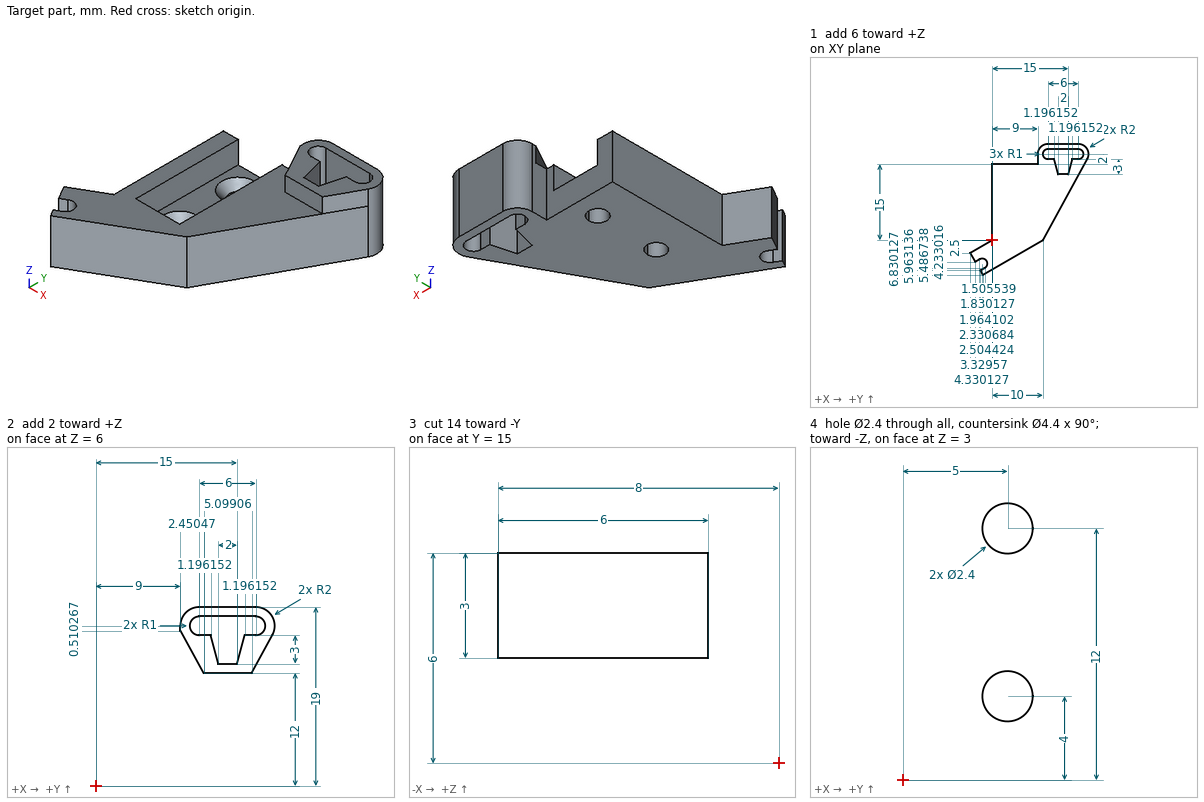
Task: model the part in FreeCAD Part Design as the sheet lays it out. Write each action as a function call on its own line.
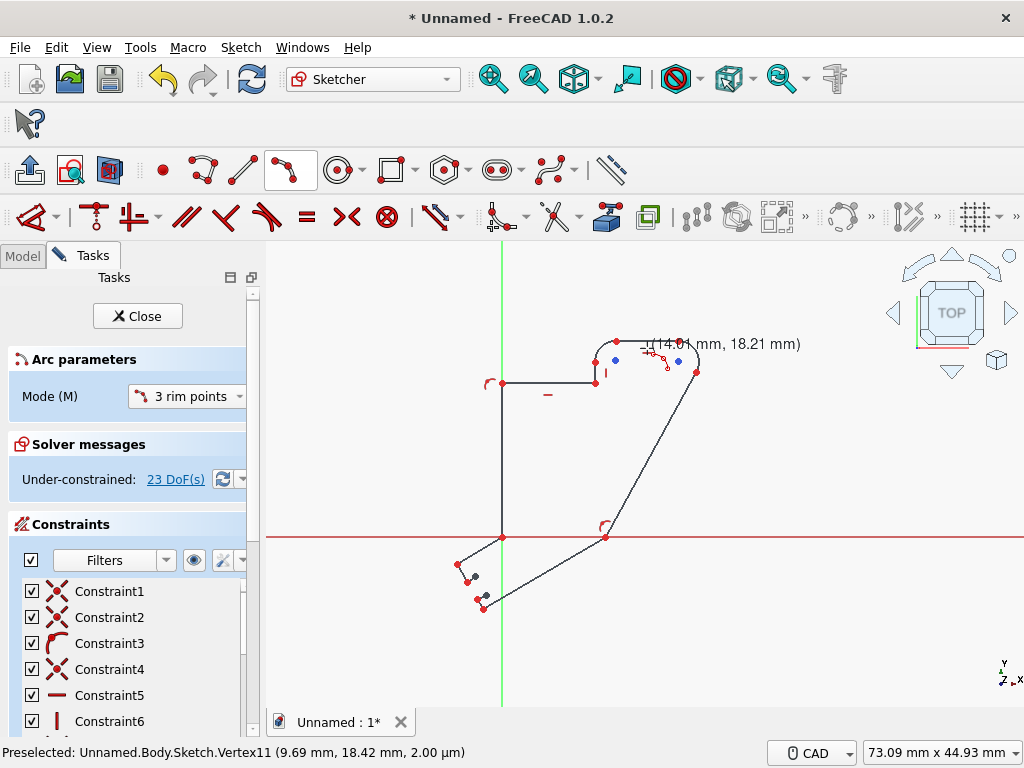
scroll(476, 576, up, 6)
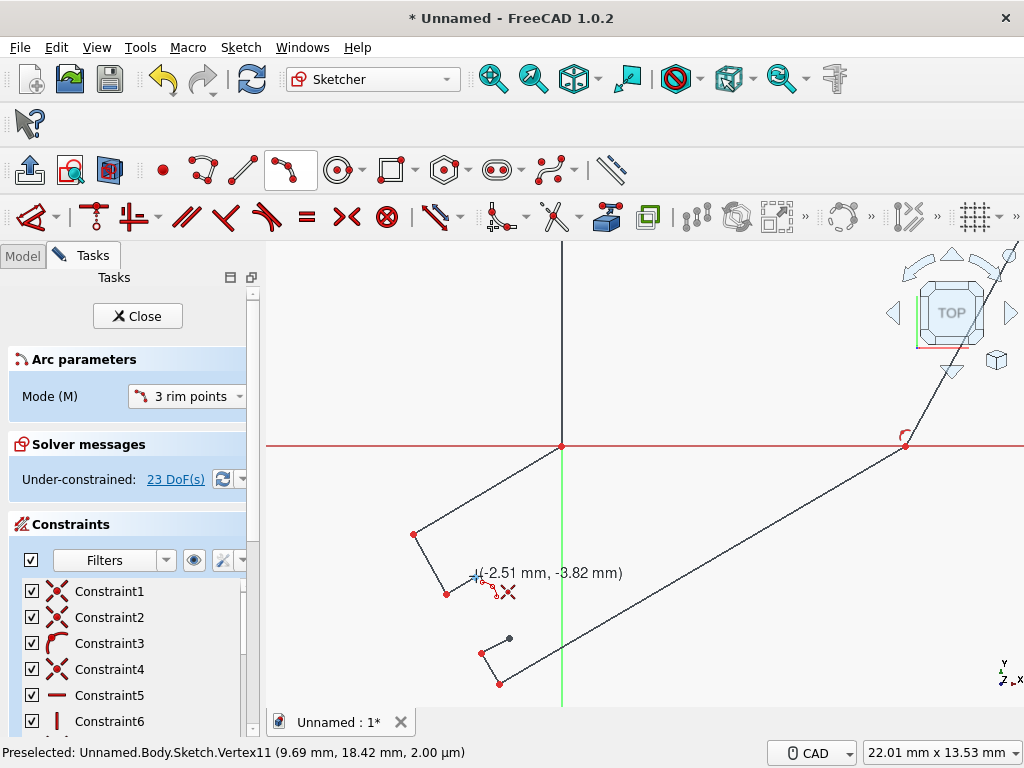
click(475, 577)
click(509, 639)
click(524, 587)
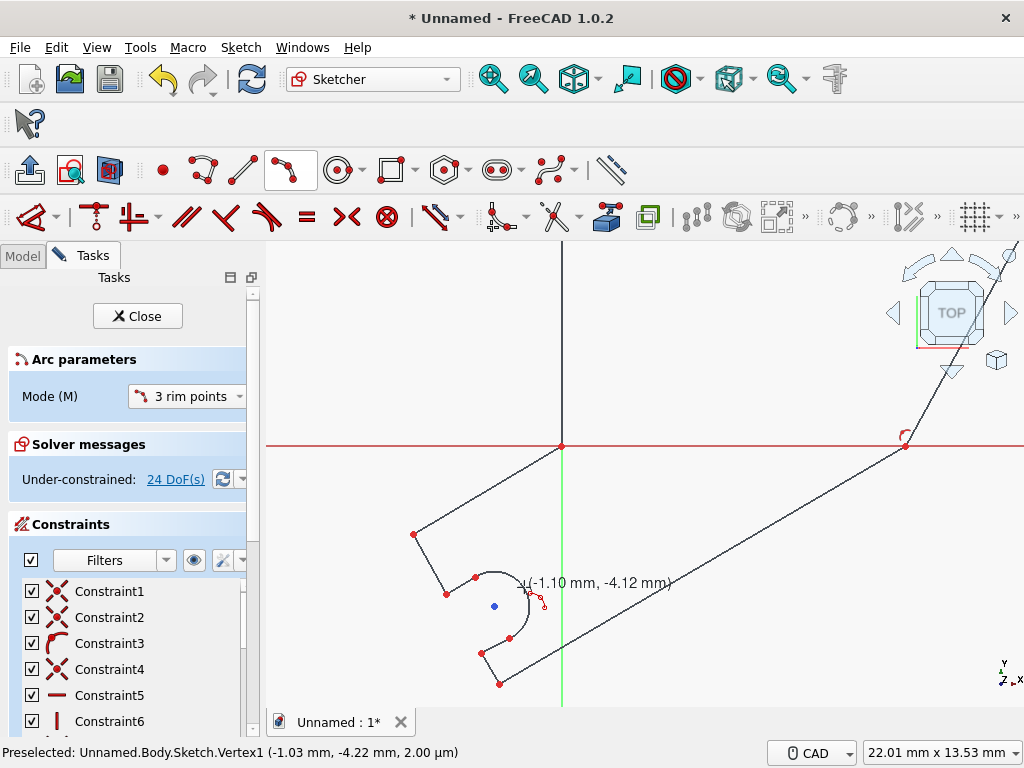
key(g)
key(l)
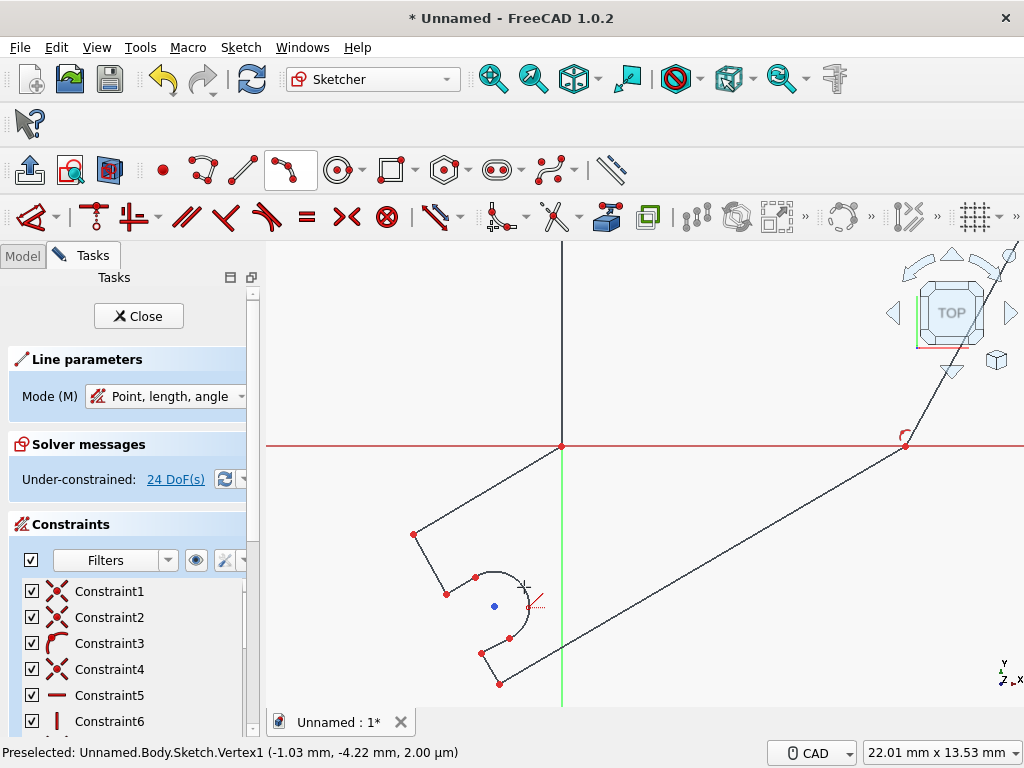
scroll(476, 576, down, 6)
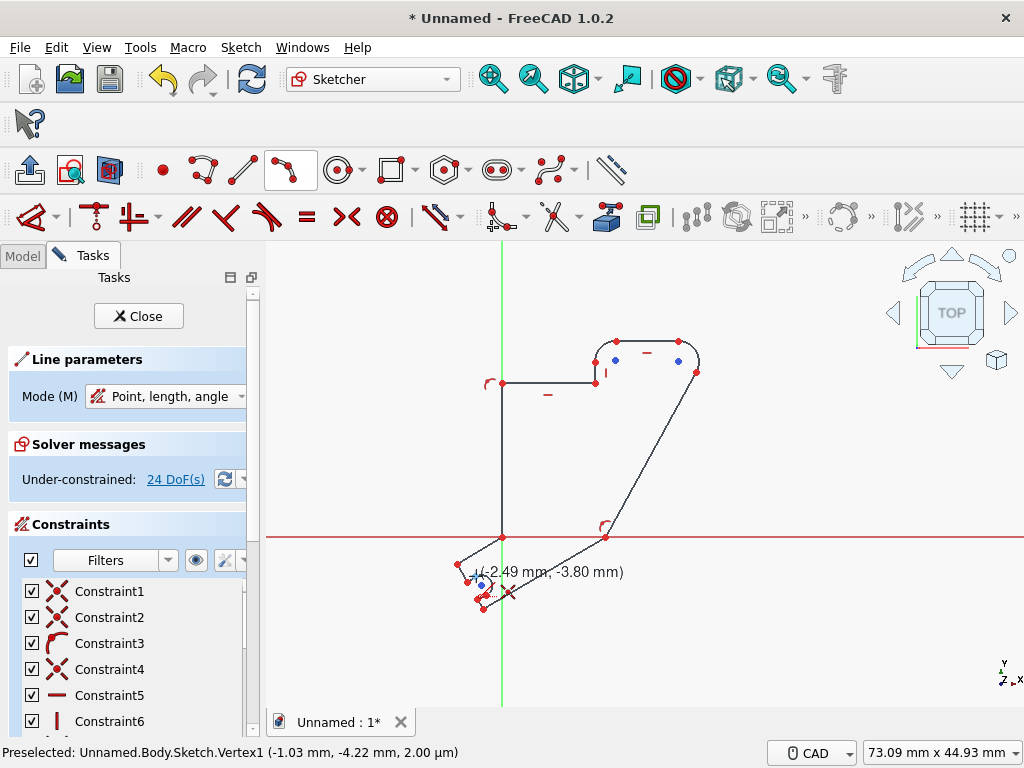
scroll(616, 351, up, 3)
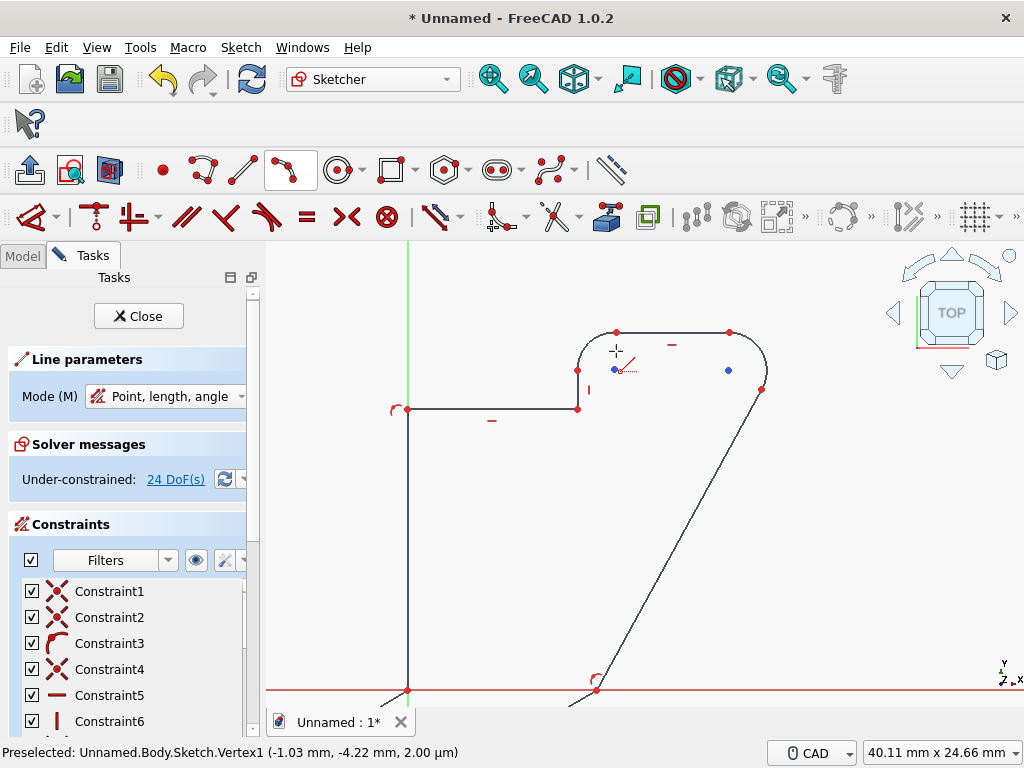
click(616, 350)
click(729, 350)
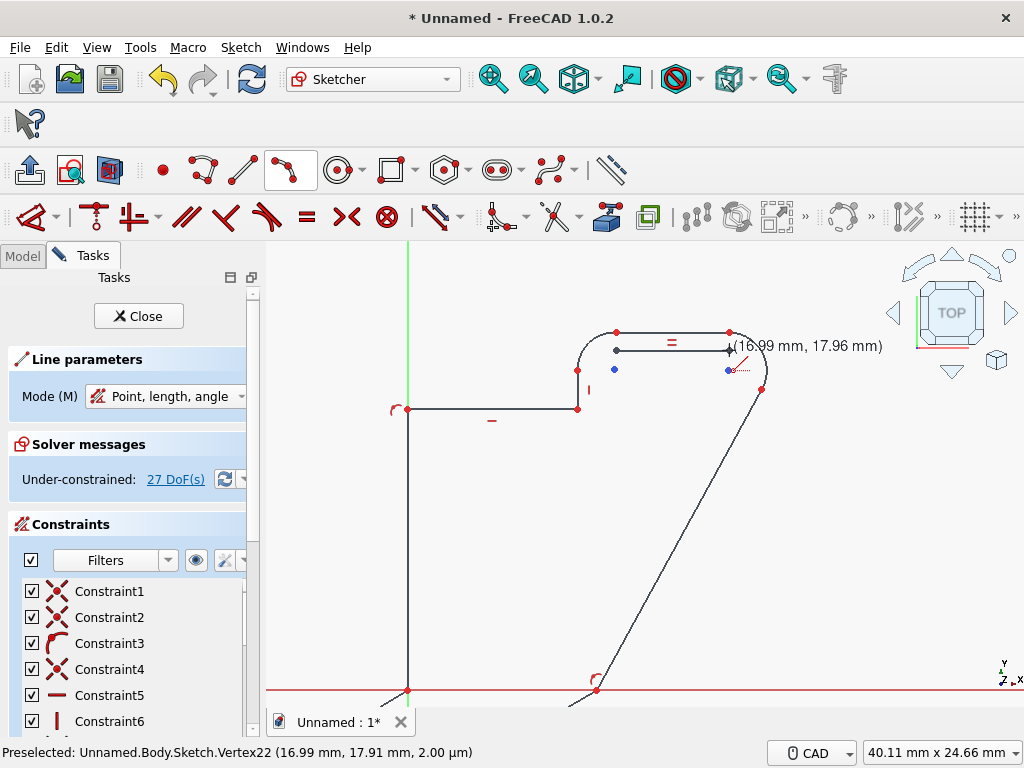
click(204, 170)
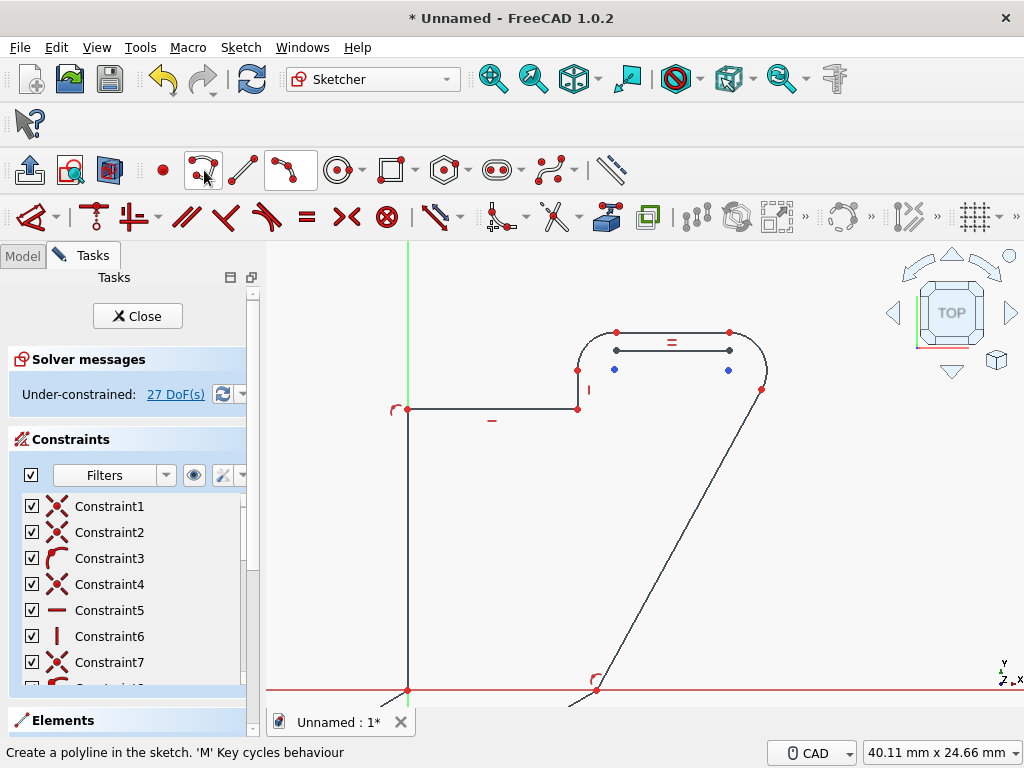
click(729, 388)
click(707, 388)
click(691, 445)
click(654, 445)
click(638, 388)
click(616, 388)
right_click(616, 388)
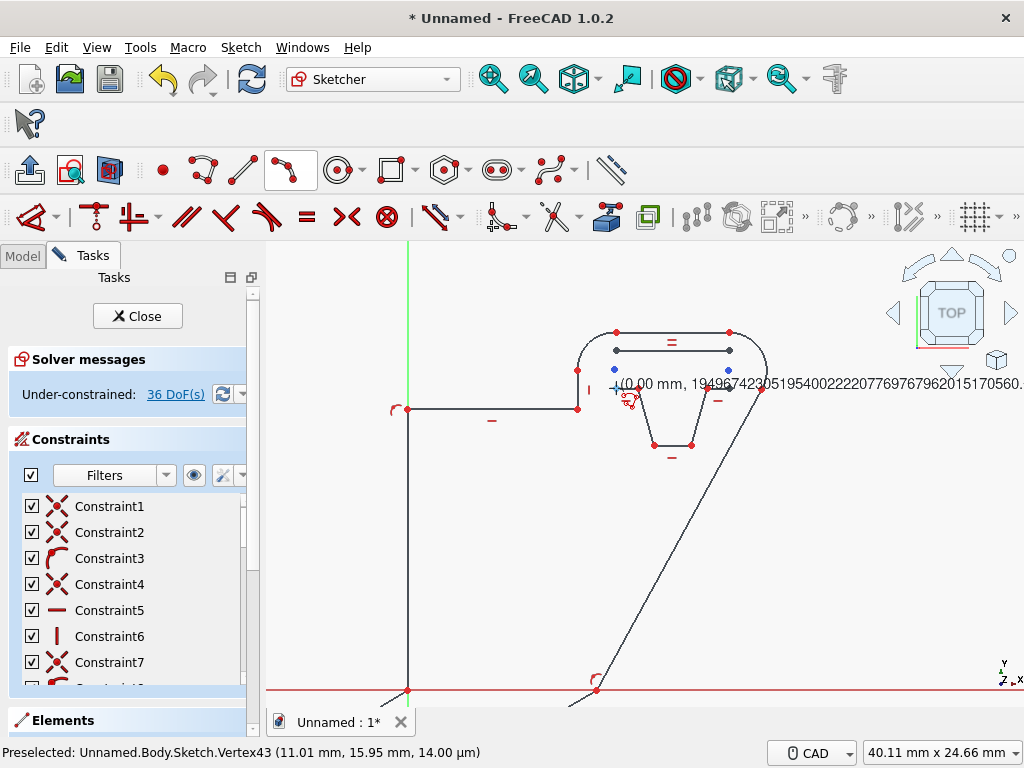
key(g)
key(3)
key(a)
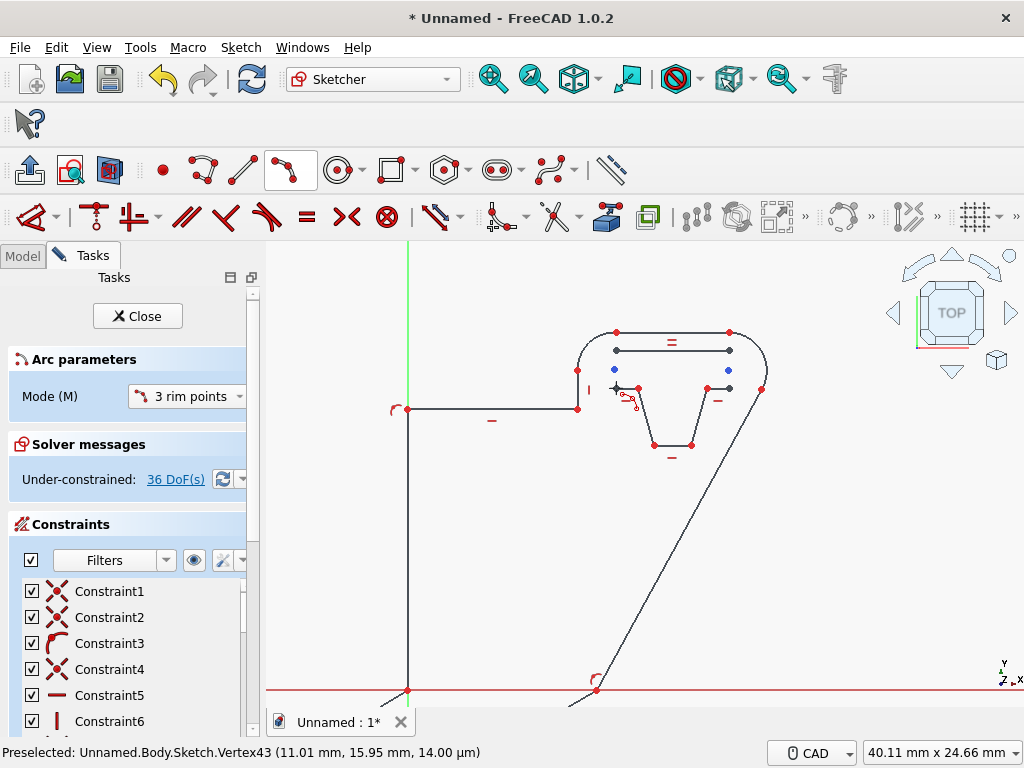
click(729, 351)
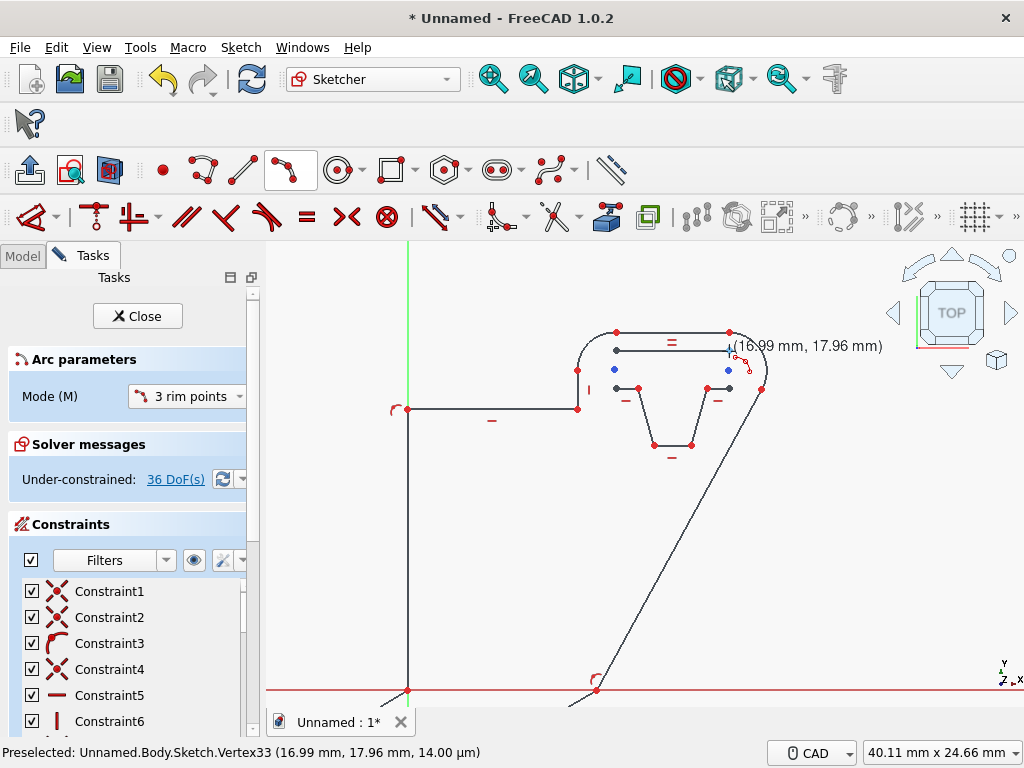
scroll(729, 388, up, 2)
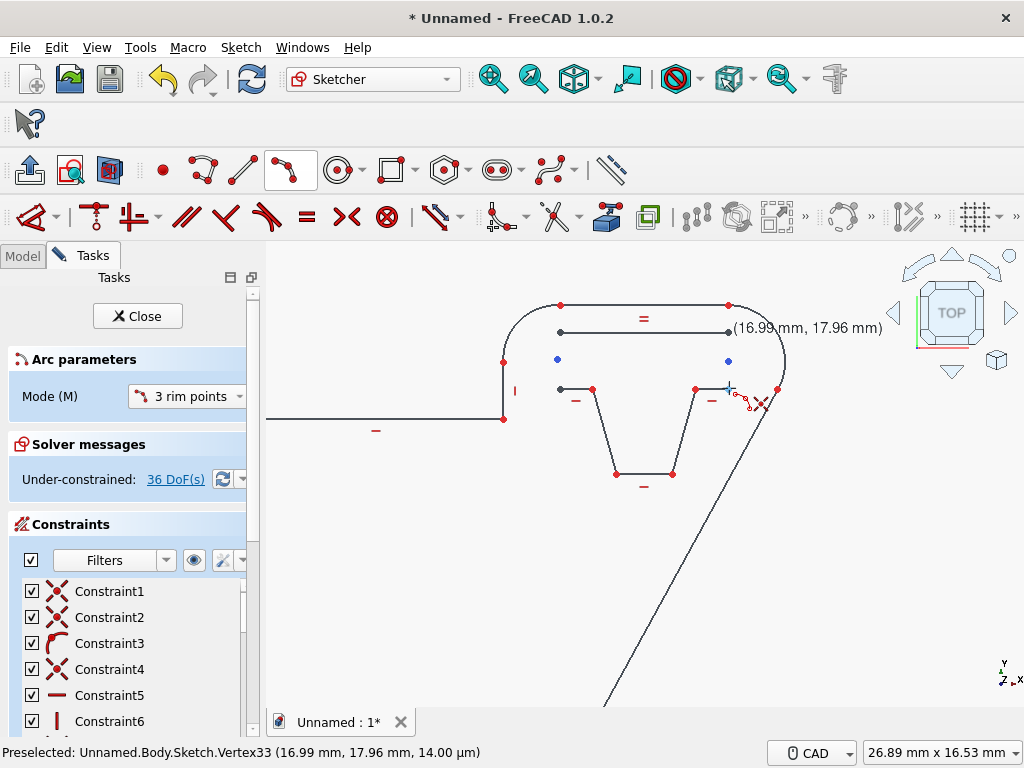
click(729, 389)
click(757, 360)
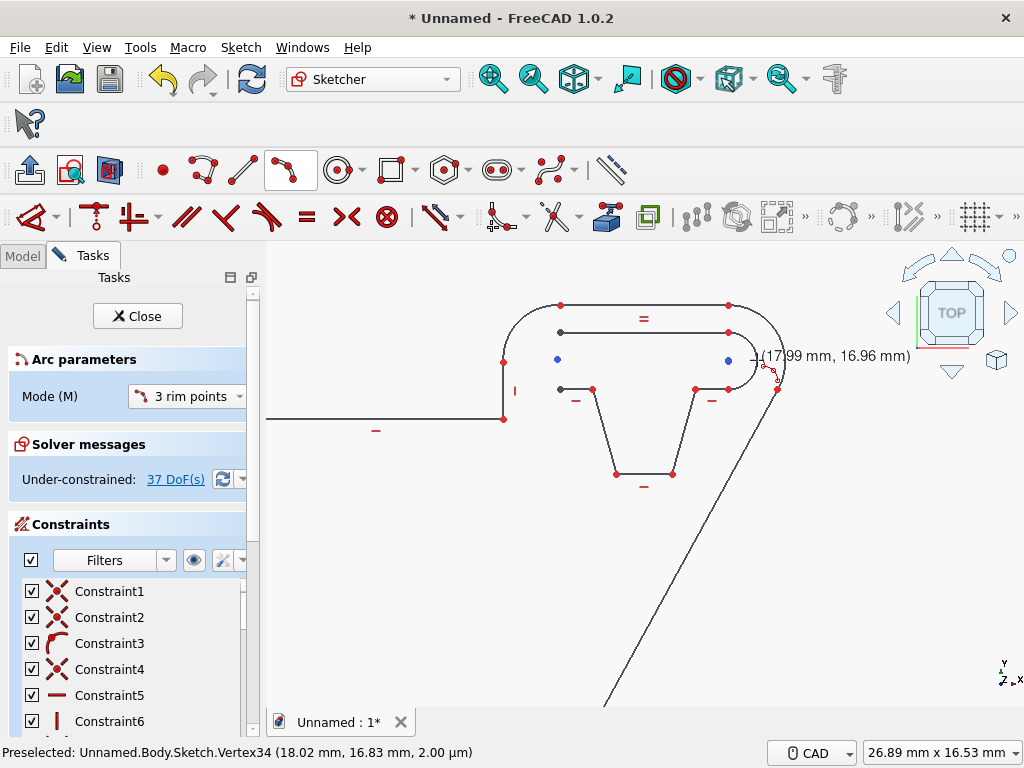
click(560, 389)
click(560, 333)
click(532, 360)
key(Escape)